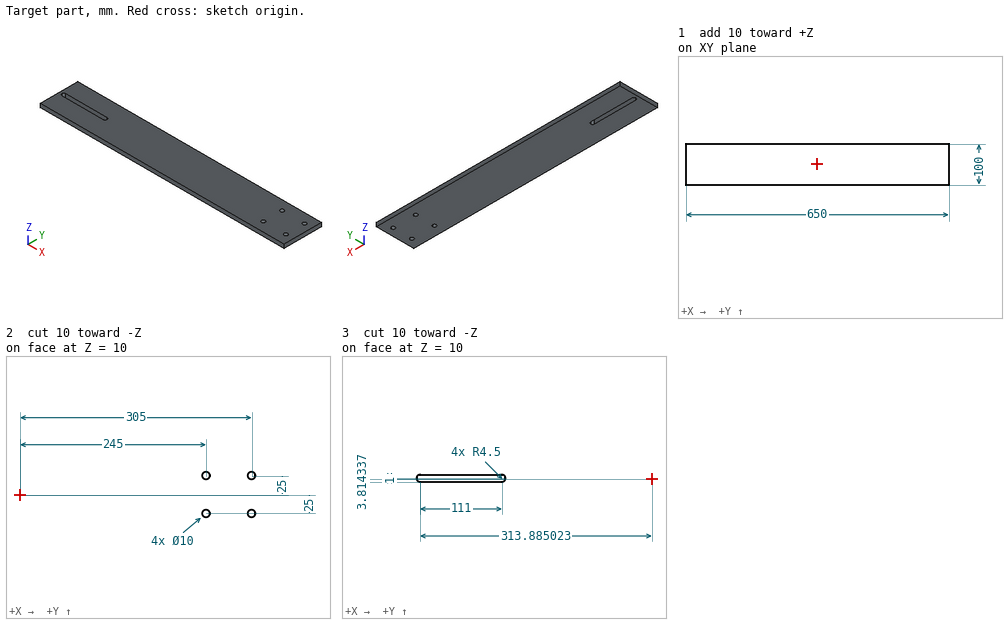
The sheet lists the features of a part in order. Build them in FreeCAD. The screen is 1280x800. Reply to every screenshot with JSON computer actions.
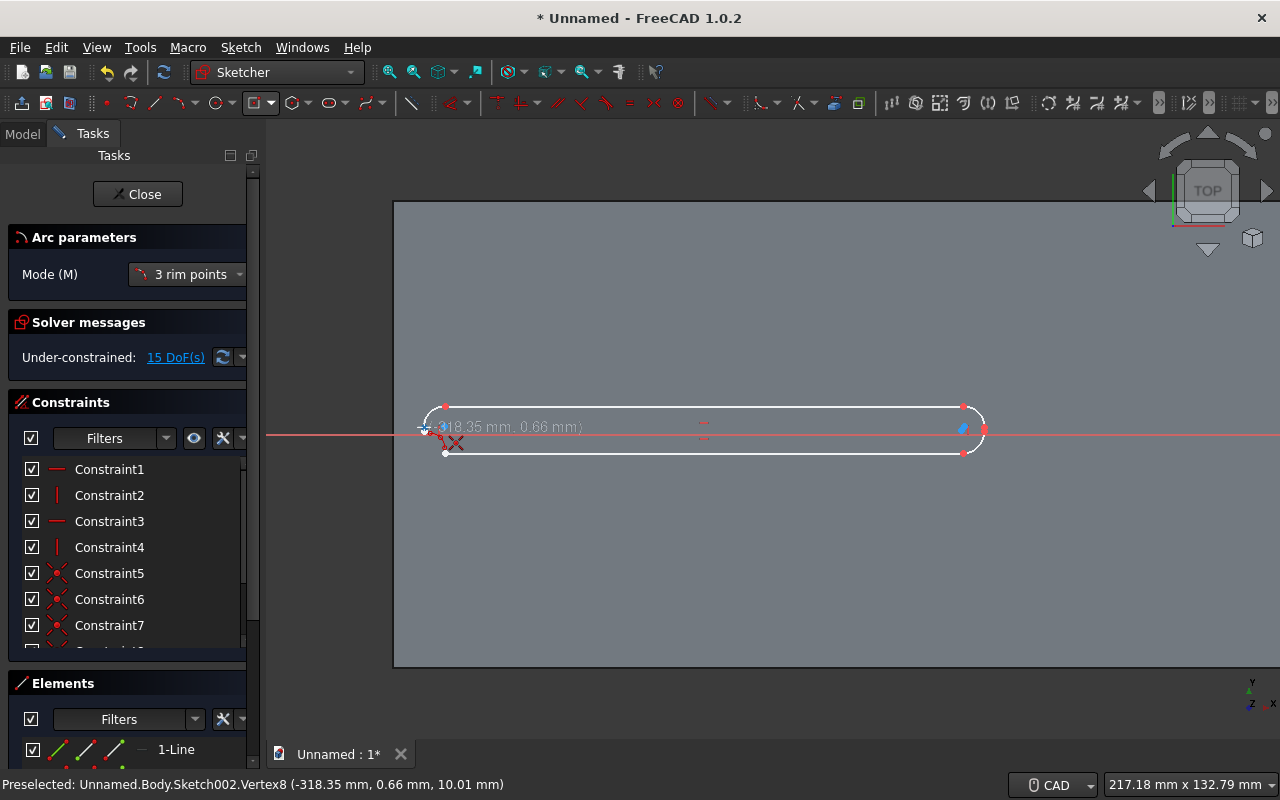
{"action": "left_click", "coordinate": [445, 454]}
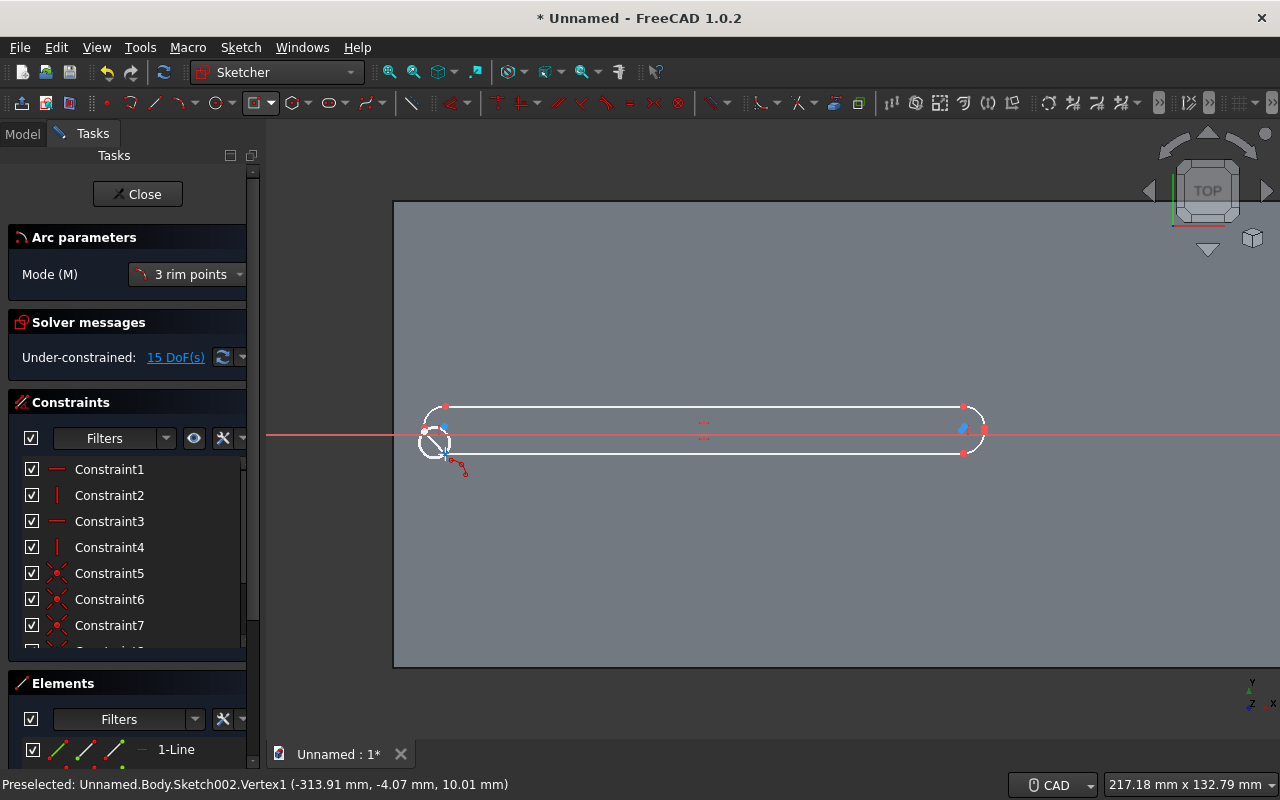
{"action": "scroll", "coordinate": [430, 446], "scroll_direction": "up", "scroll_amount": 5}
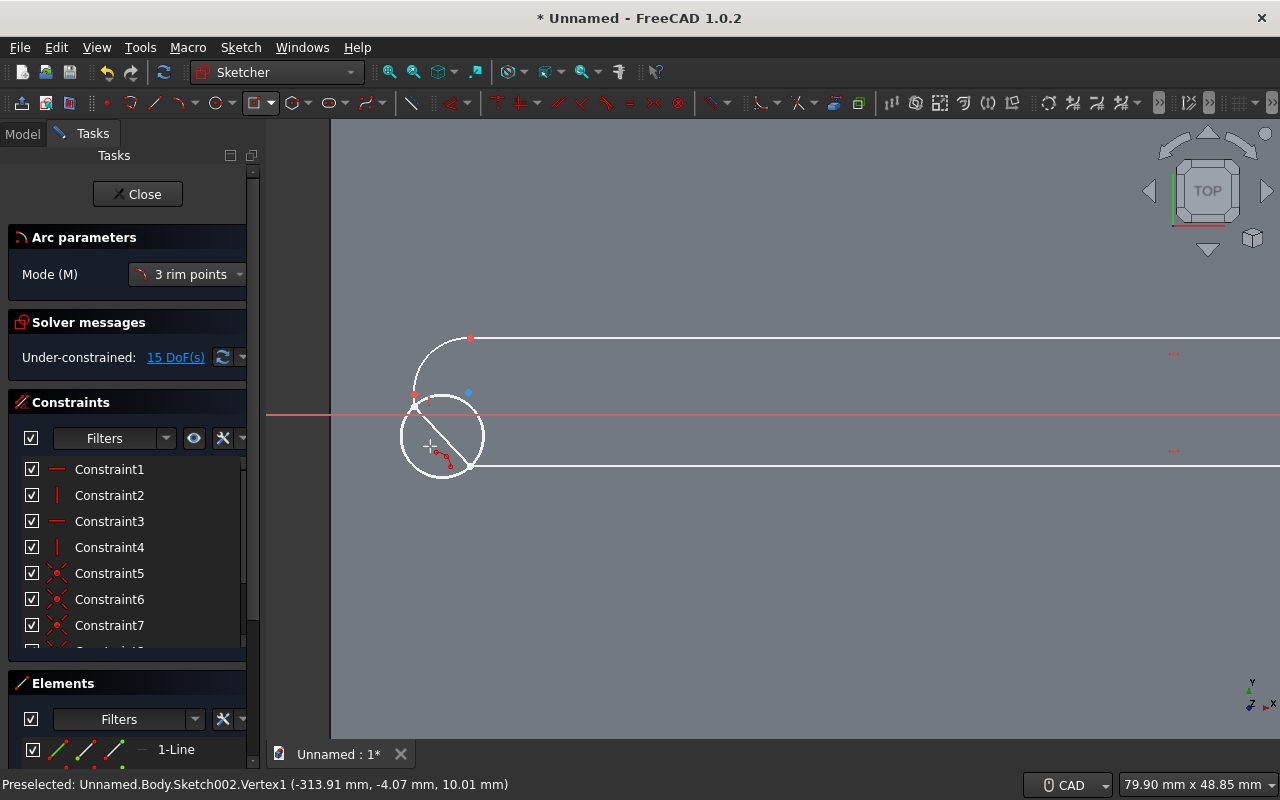
{"action": "left_click", "coordinate": [430, 446]}
{"action": "key", "text": "Escape"}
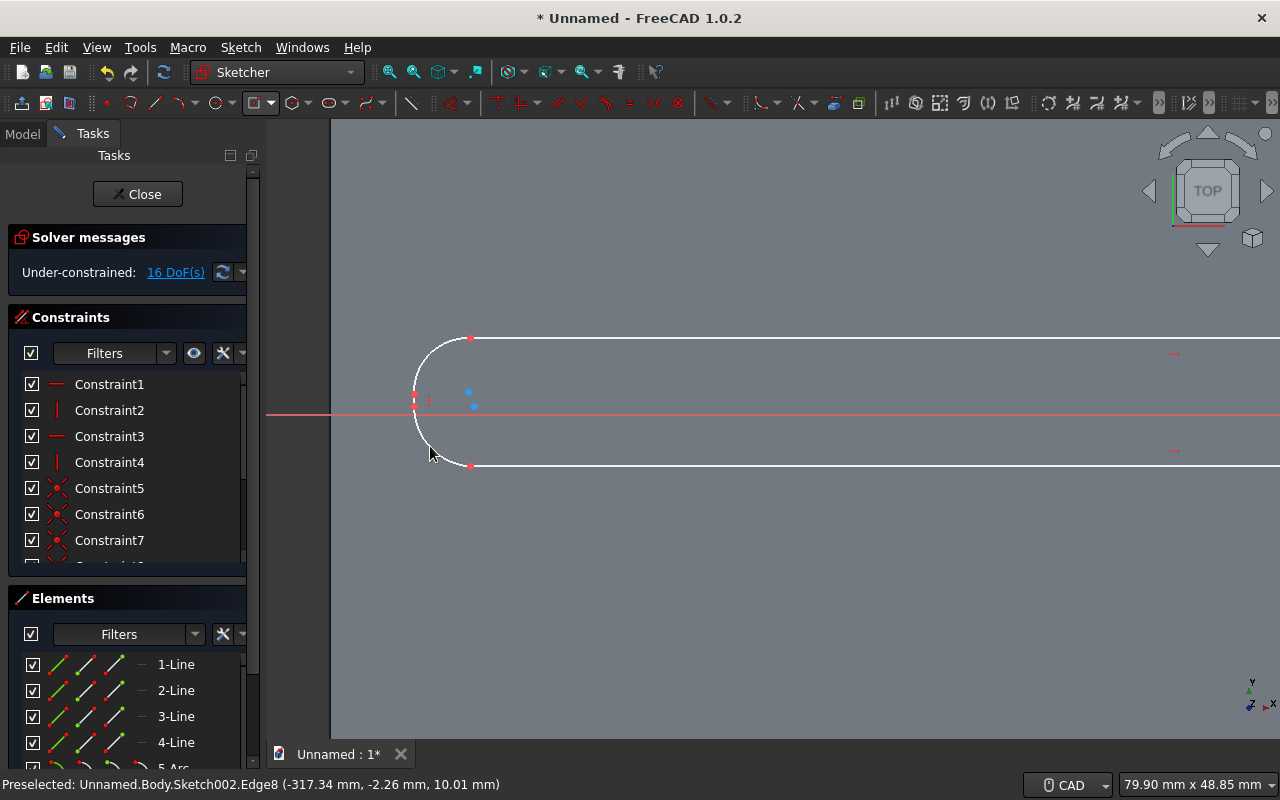
{"action": "left_click", "coordinate": [893, 466]}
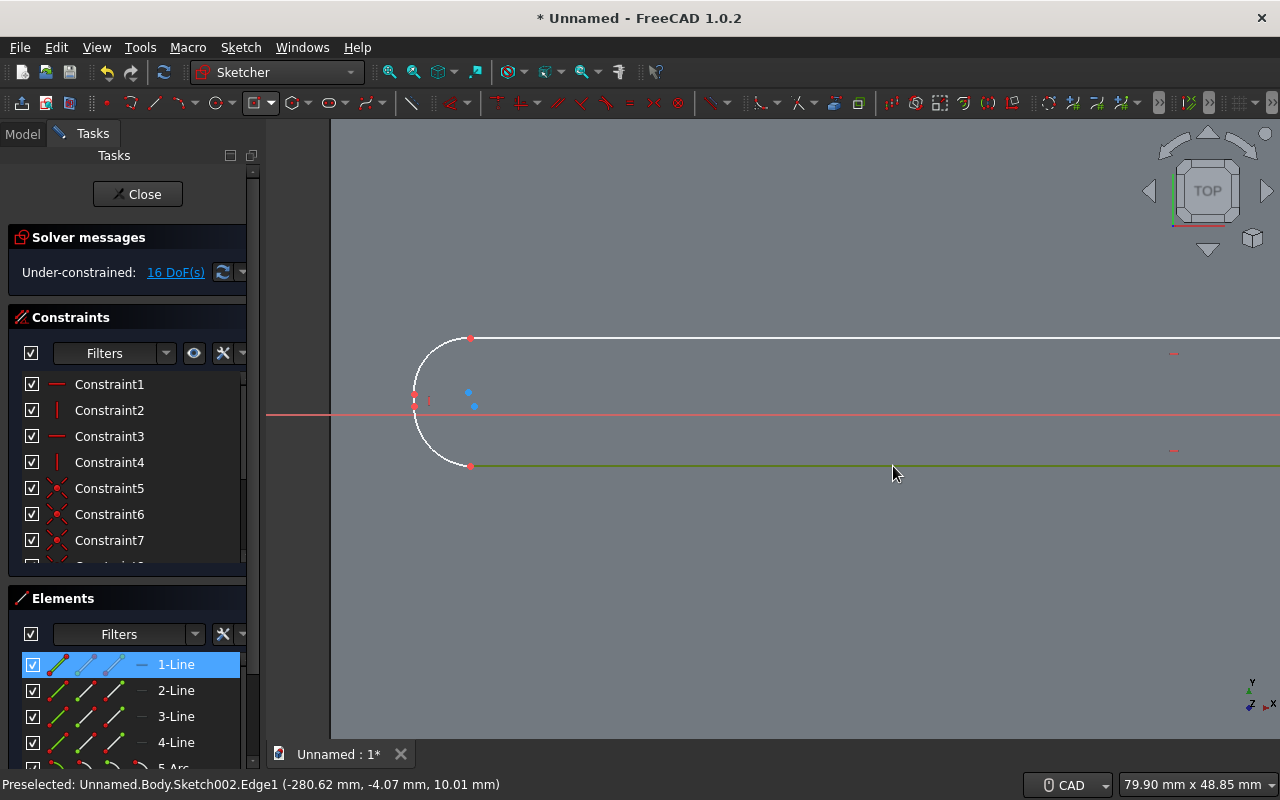
{"action": "scroll", "coordinate": [431, 446], "scroll_direction": "down", "scroll_amount": 5}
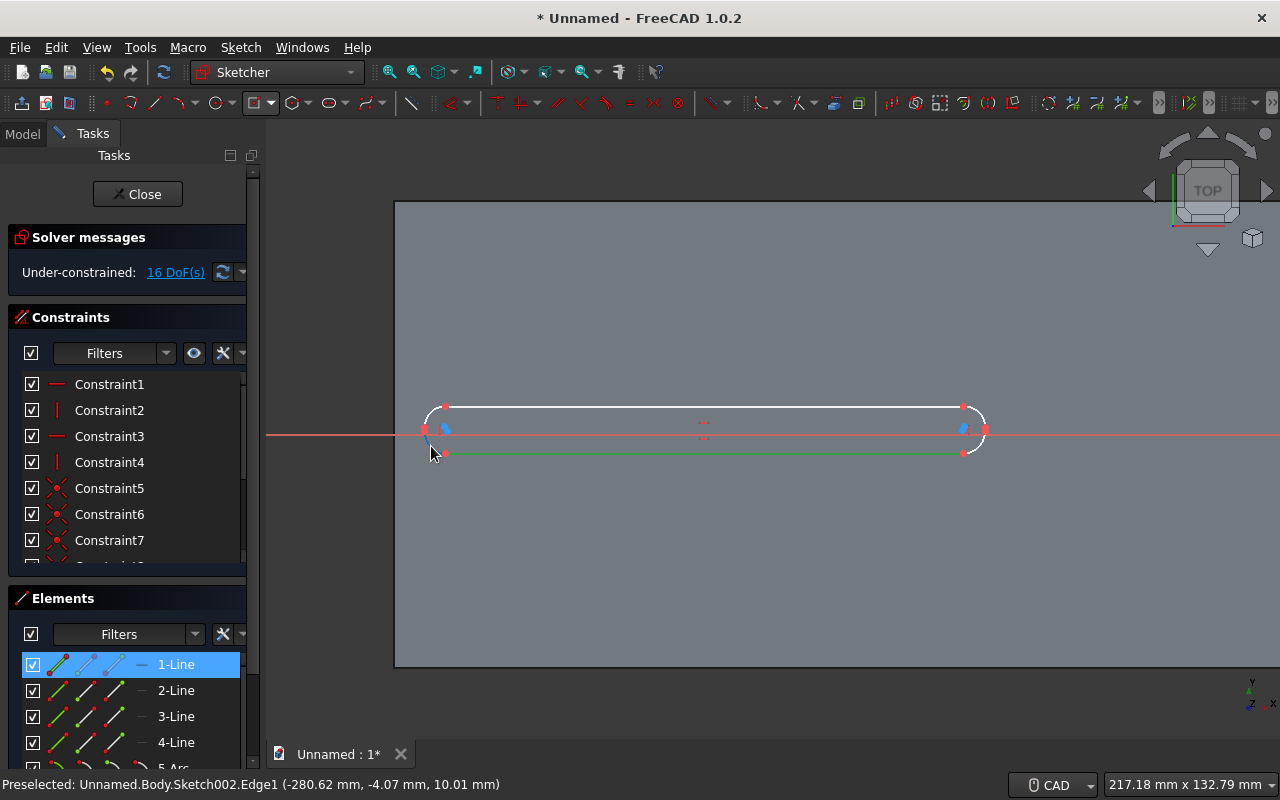
{"action": "scroll", "coordinate": [973, 451], "scroll_direction": "up", "scroll_amount": 2}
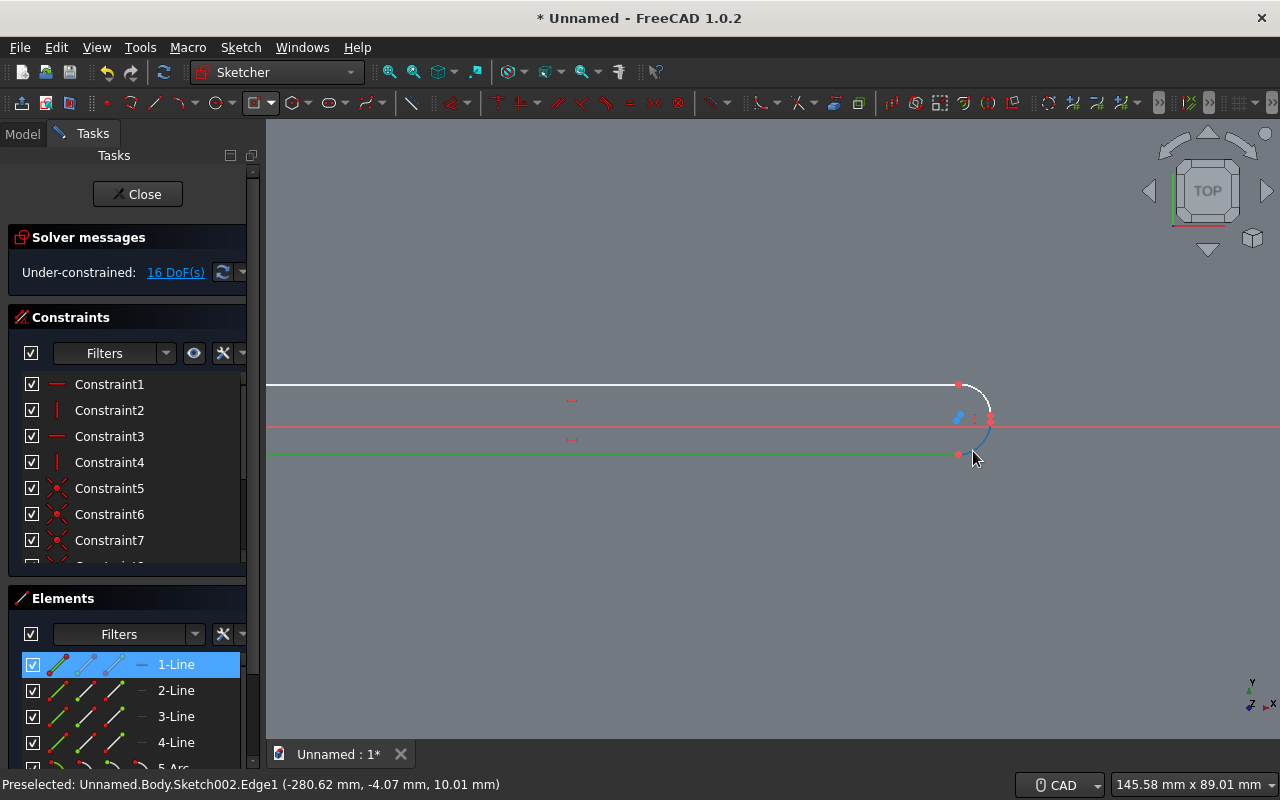
{"action": "left_click", "coordinate": [973, 451]}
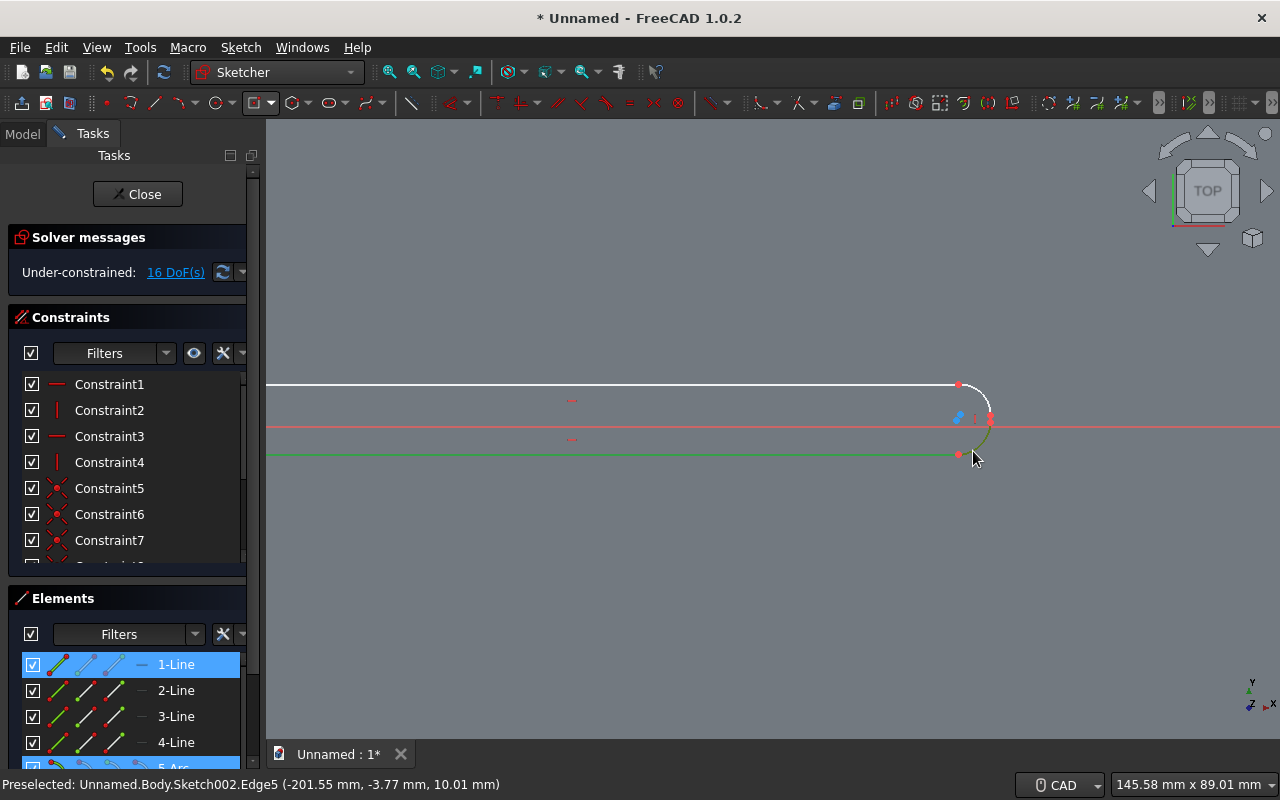
{"action": "key", "text": "t"}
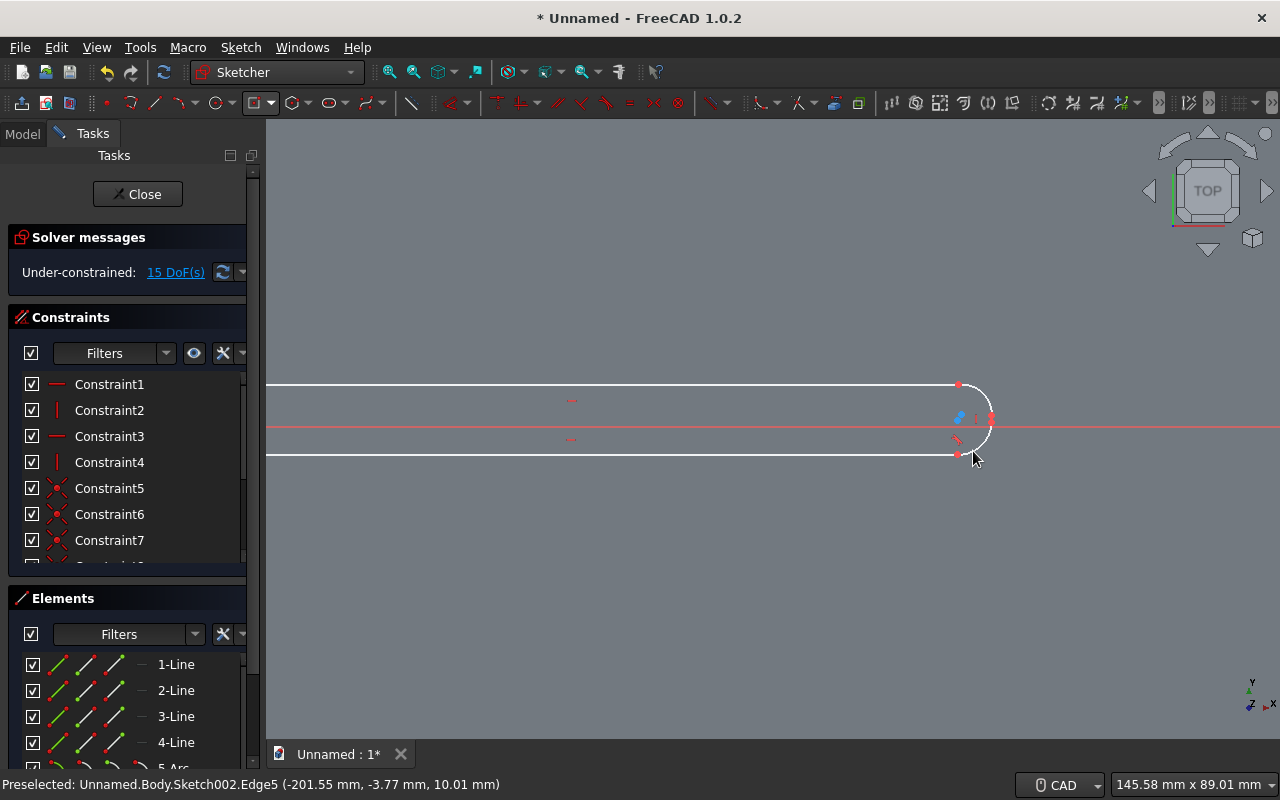
{"action": "left_click", "coordinate": [417, 455]}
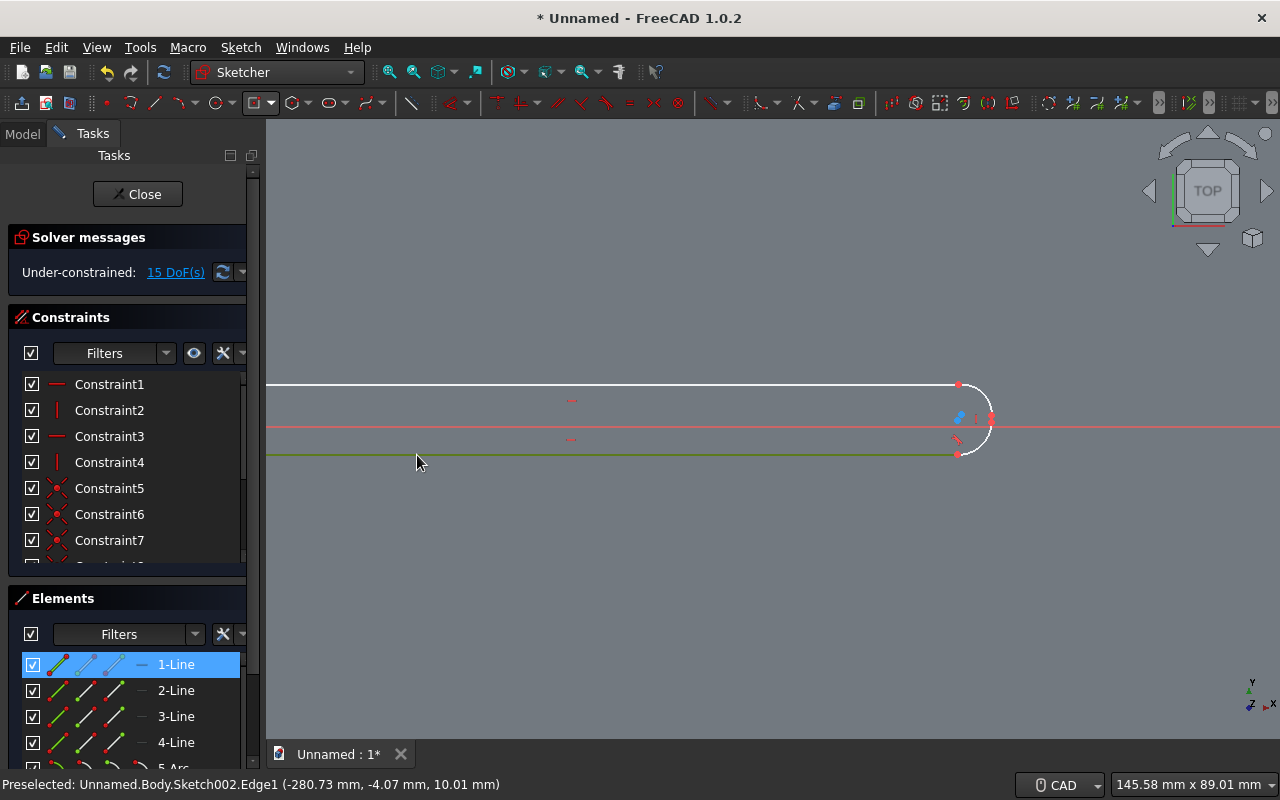
{"action": "scroll", "coordinate": [973, 451], "scroll_direction": "down", "scroll_amount": 2}